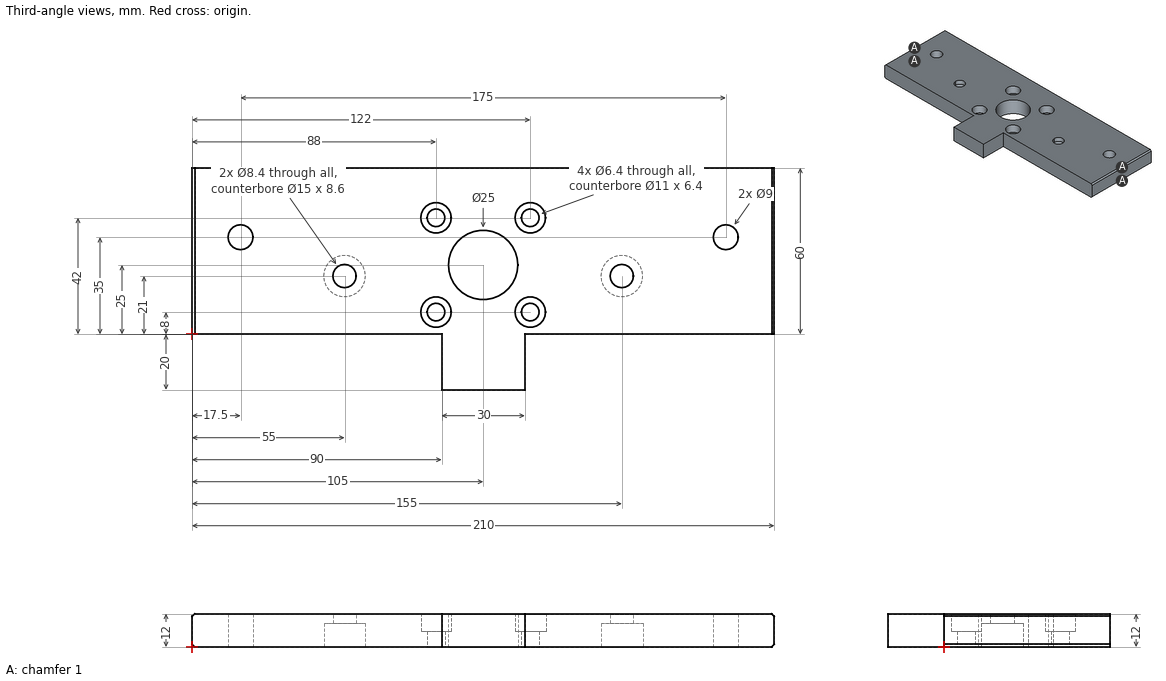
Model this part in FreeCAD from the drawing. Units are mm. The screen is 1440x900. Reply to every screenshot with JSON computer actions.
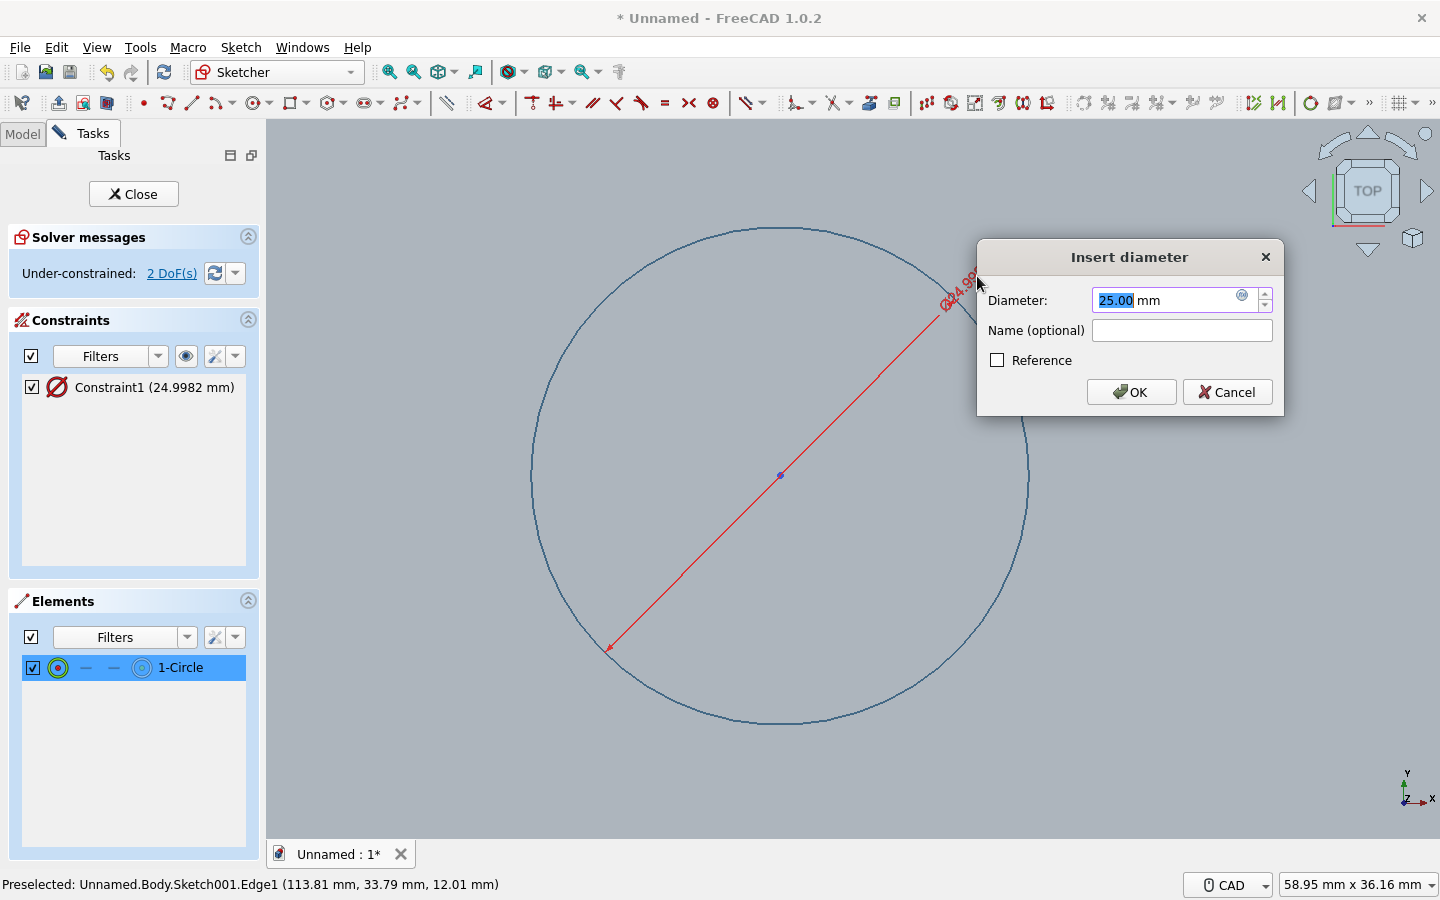
{"action": "type", "text": "25"}
{"action": "key", "text": "Return"}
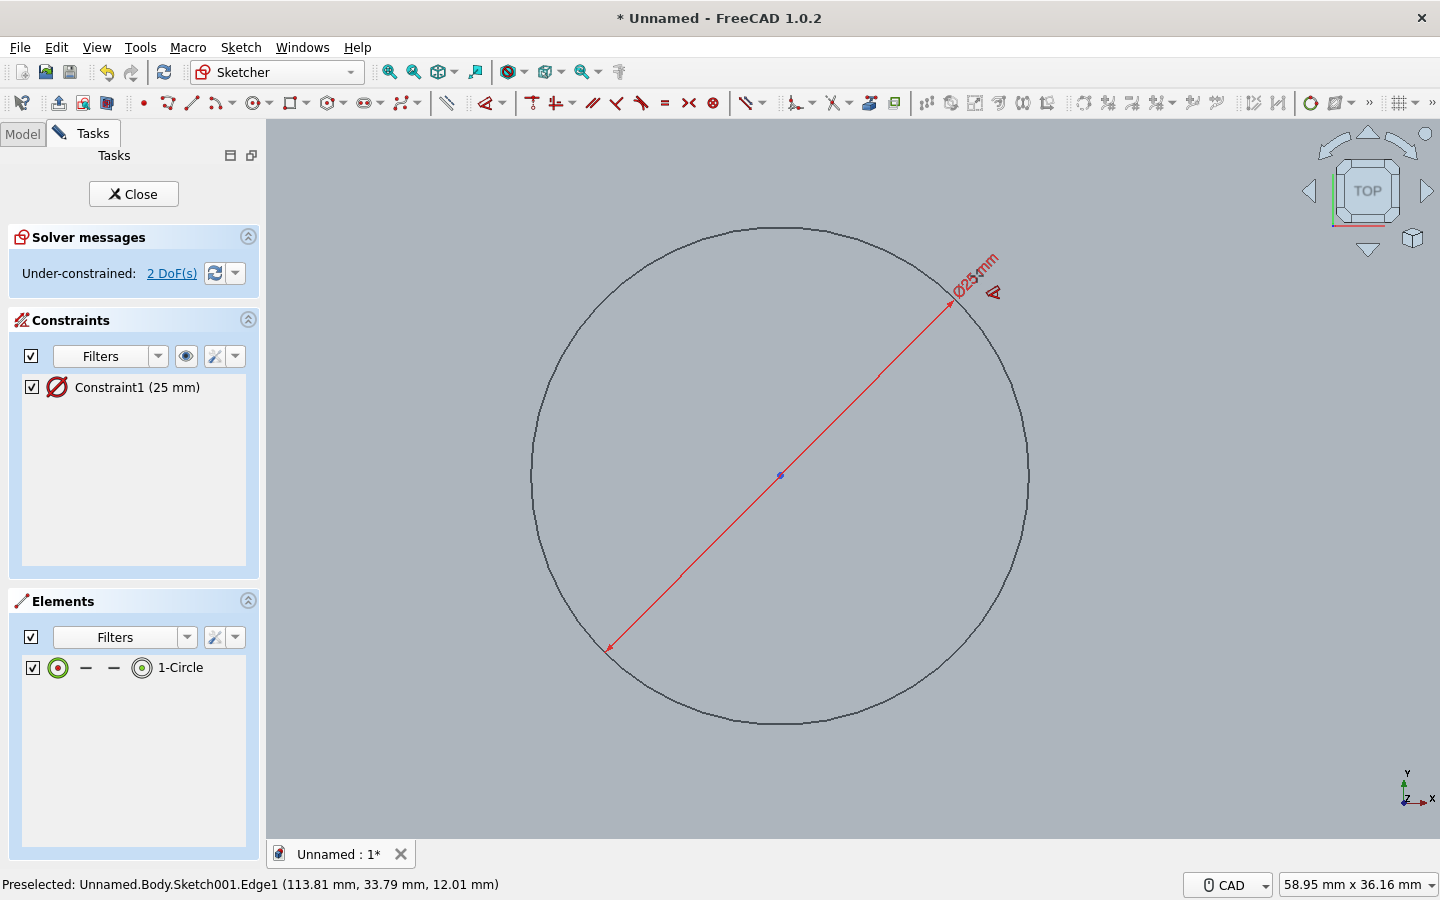
{"action": "left_click", "coordinate": [780, 476]}
{"action": "left_click", "coordinate": [814, 643]}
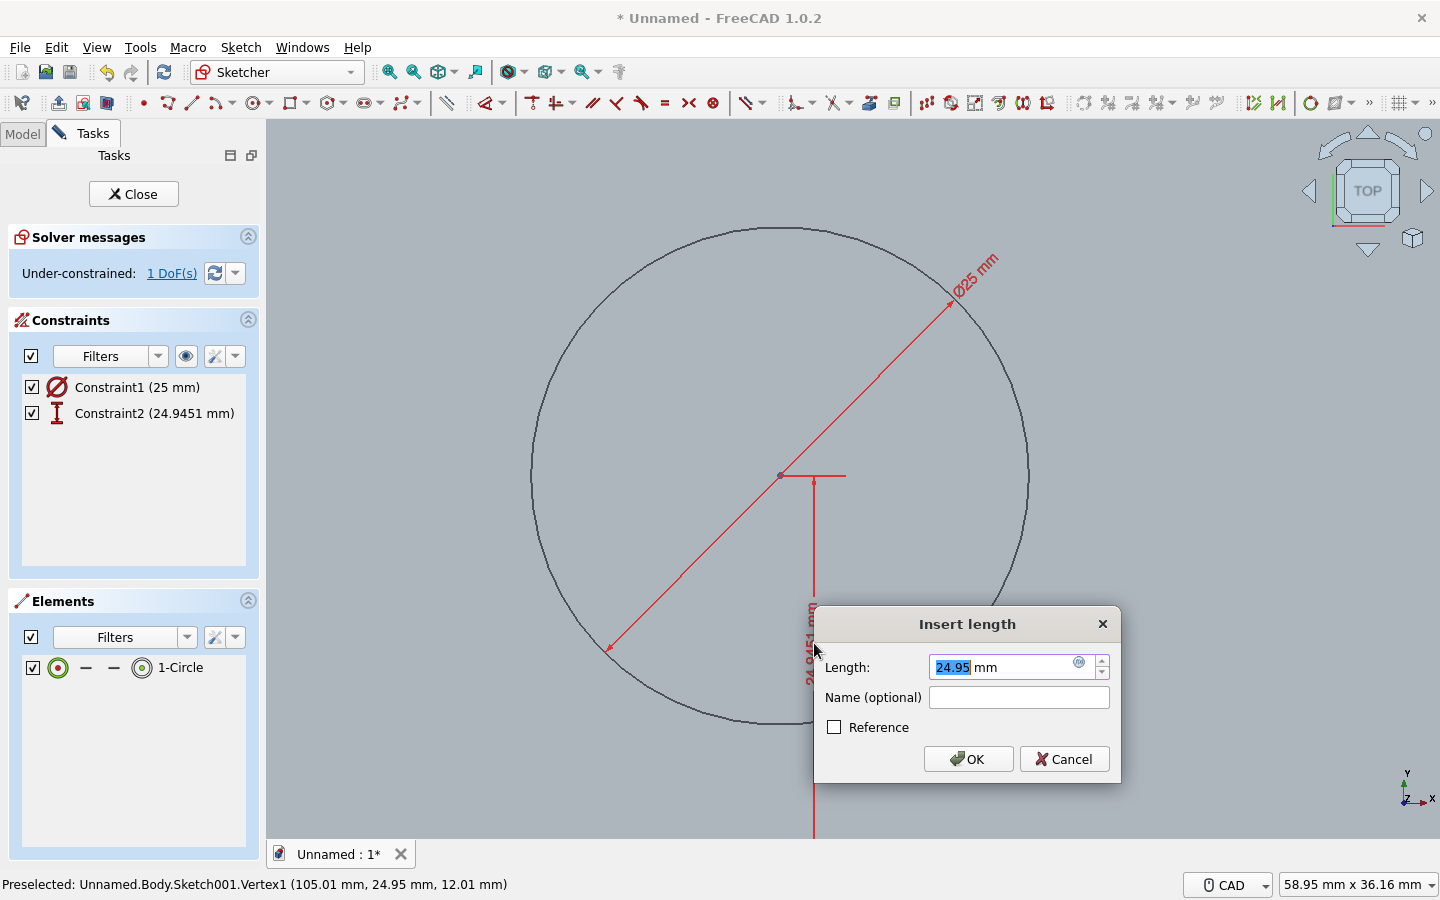
{"action": "type", "text": "25"}
{"action": "key", "text": "Return"}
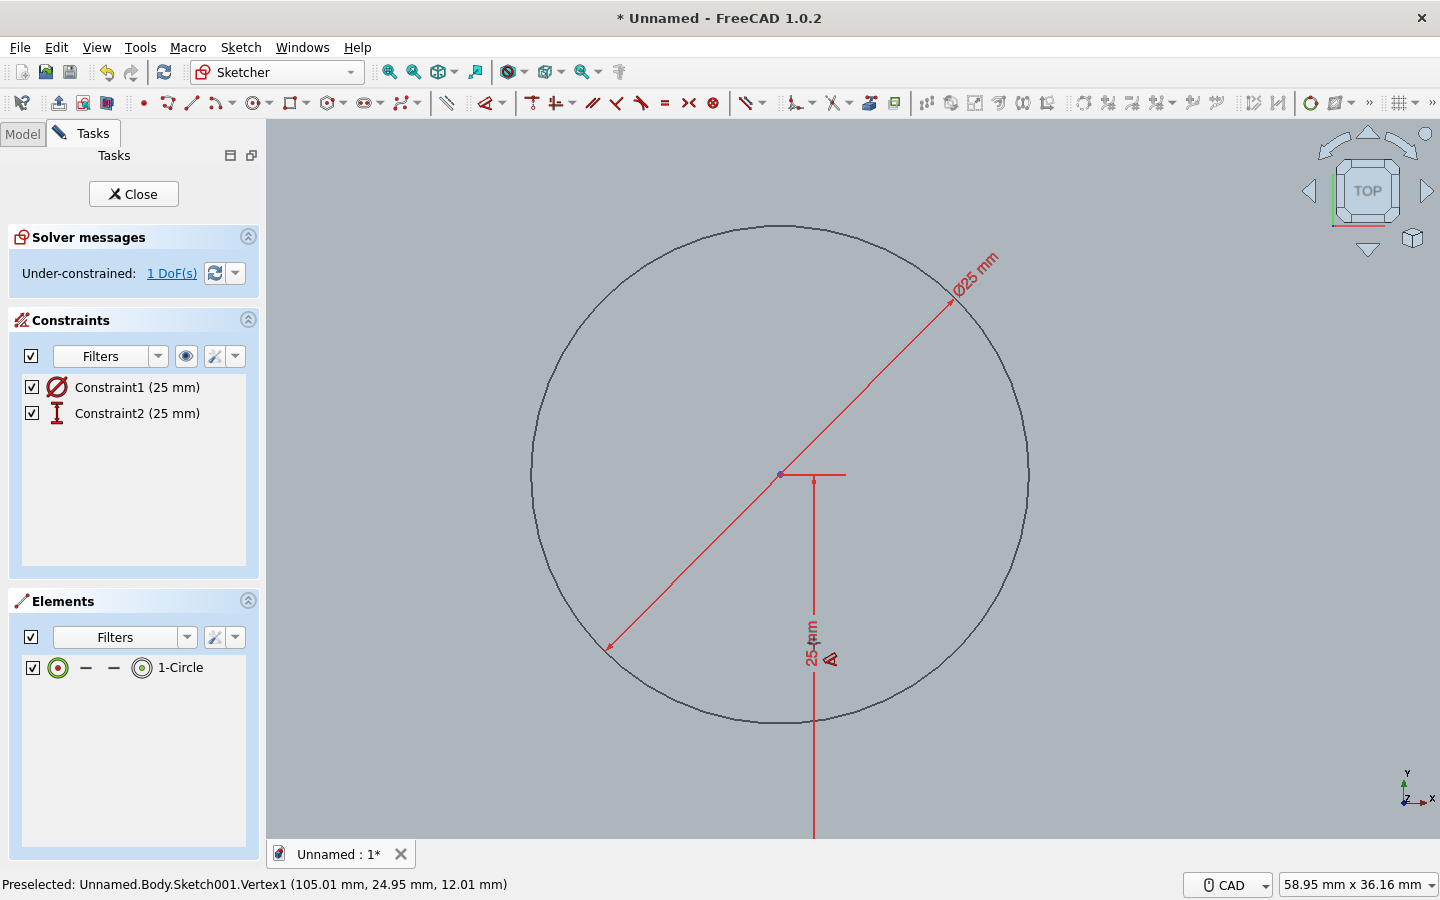
{"action": "left_click", "coordinate": [780, 475]}
{"action": "left_click", "coordinate": [425, 441]}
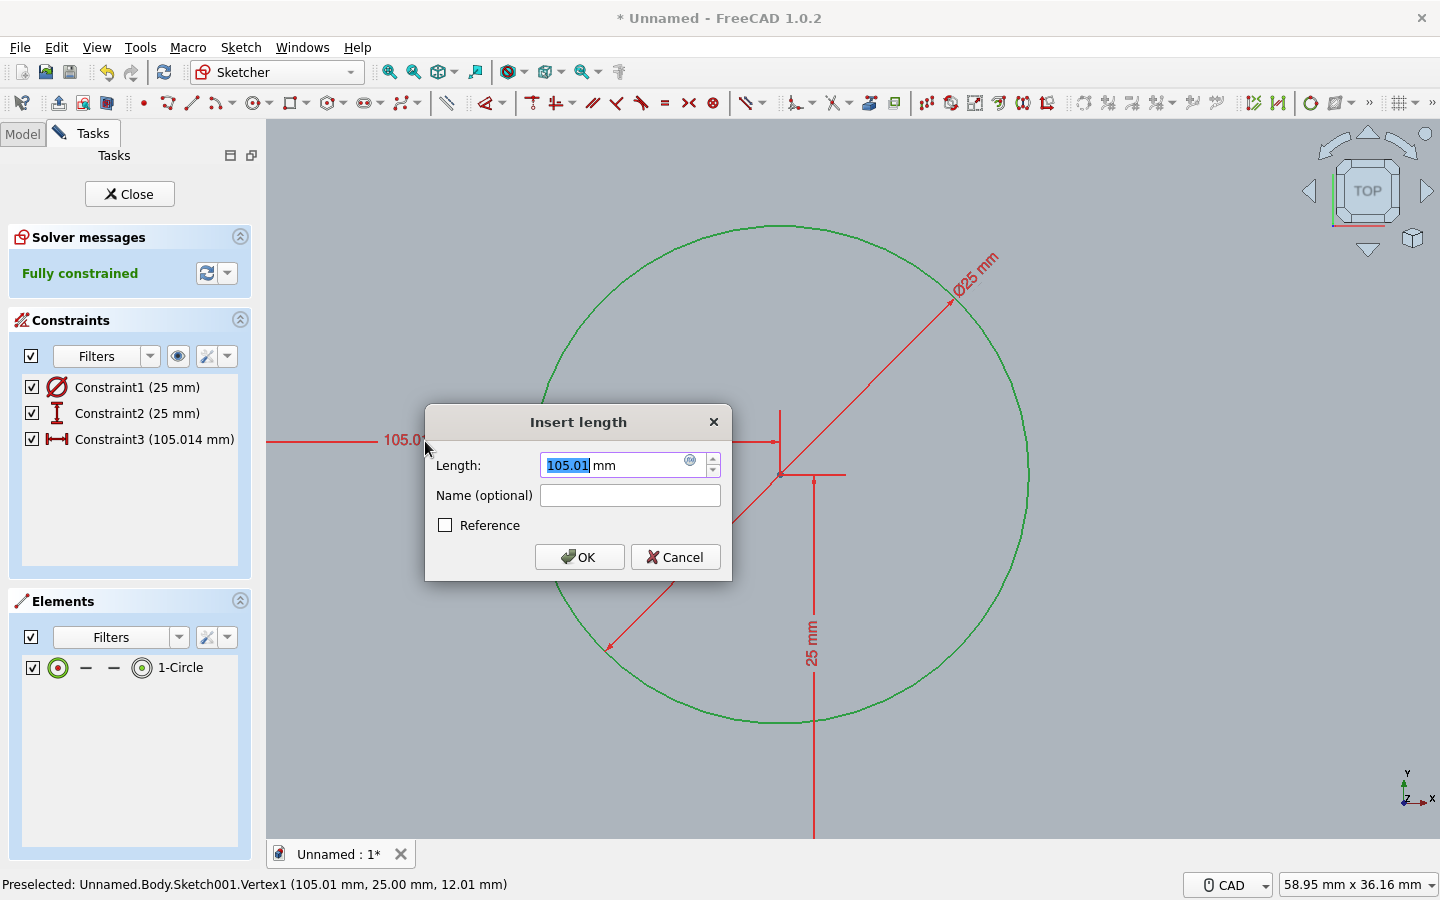
{"action": "type", "text": "105"}
{"action": "key", "text": "Return"}
{"action": "key", "text": "Escape"}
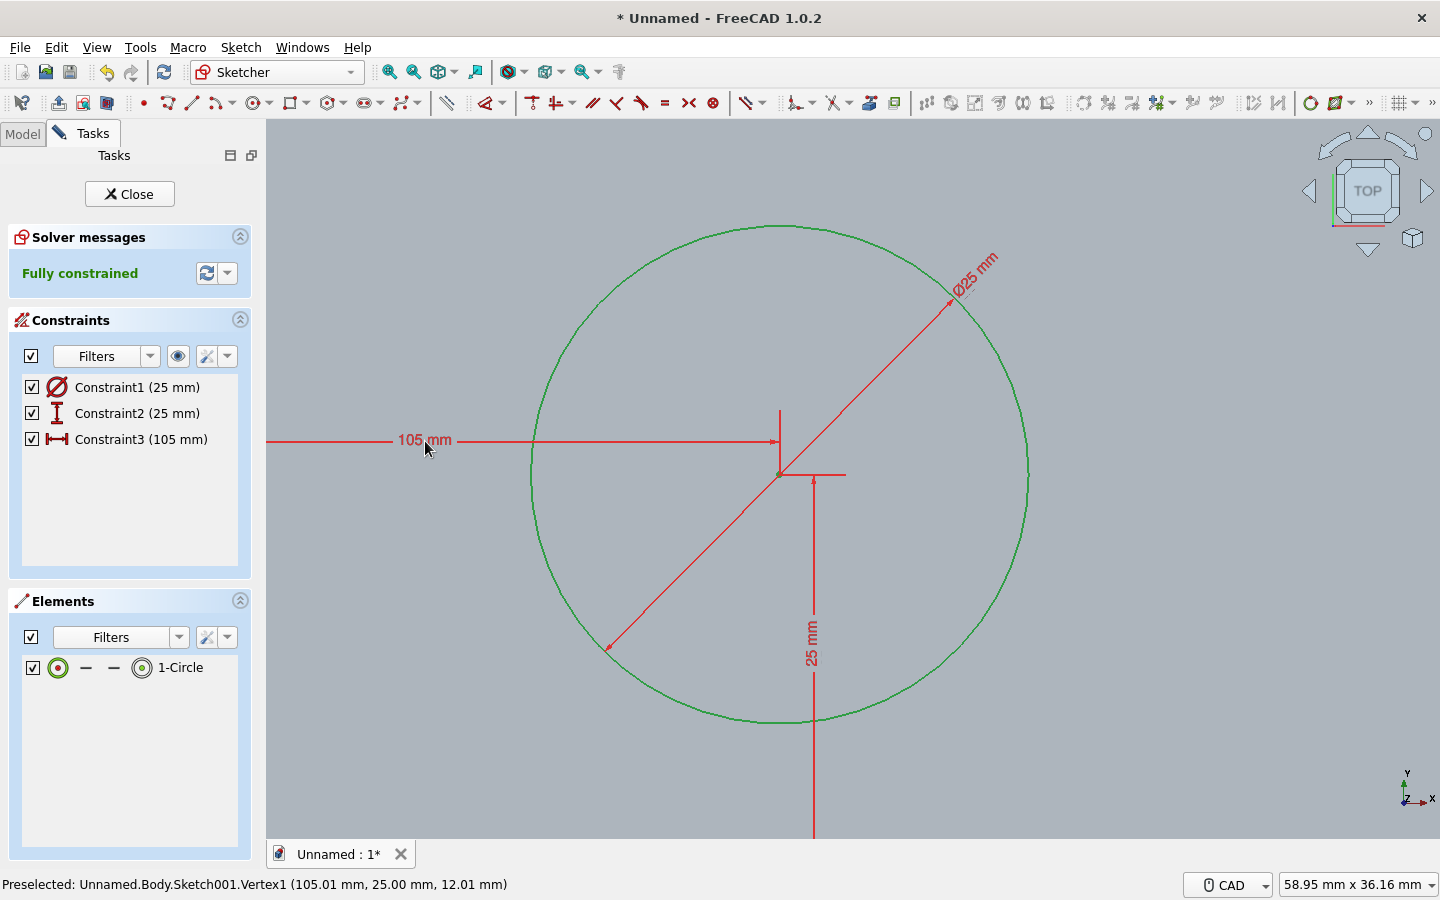
{"action": "left_click", "coordinate": [130, 194]}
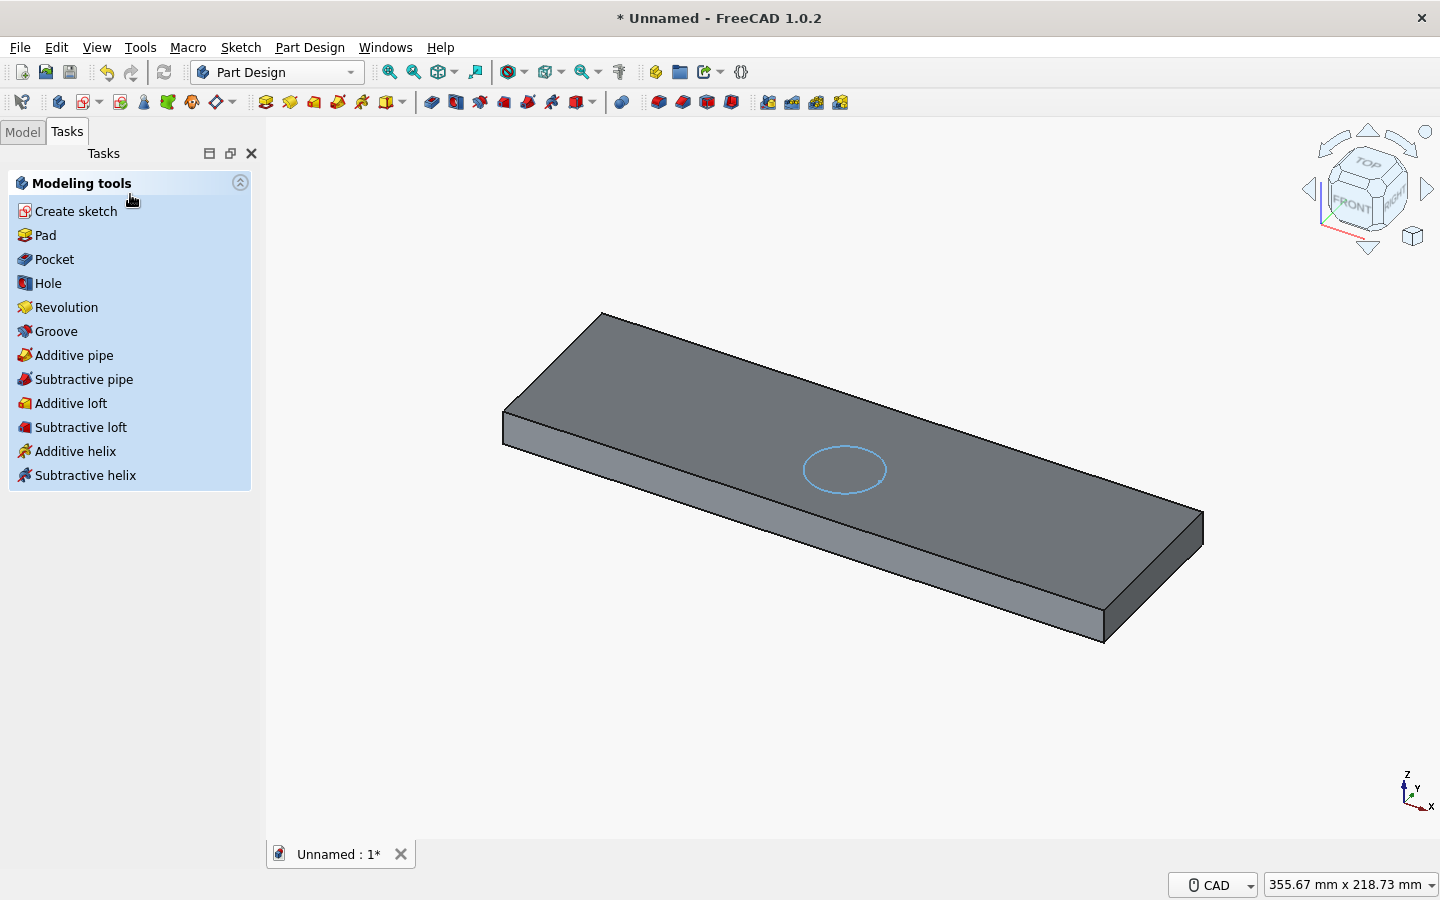
{"action": "left_click", "coordinate": [432, 102]}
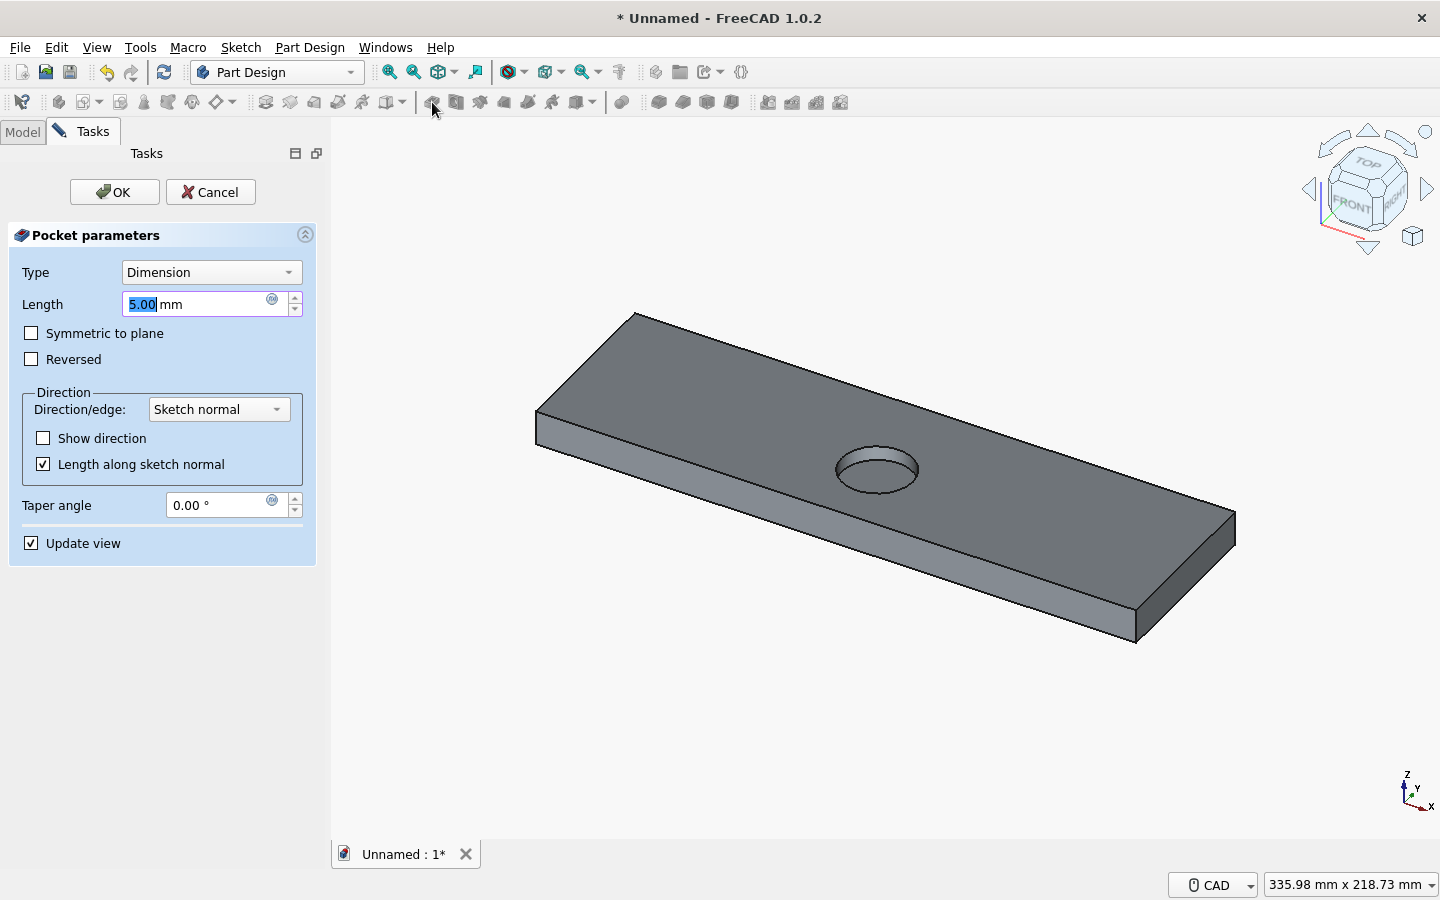
{"action": "type", "text": "12"}
{"action": "key", "text": "Tab"}